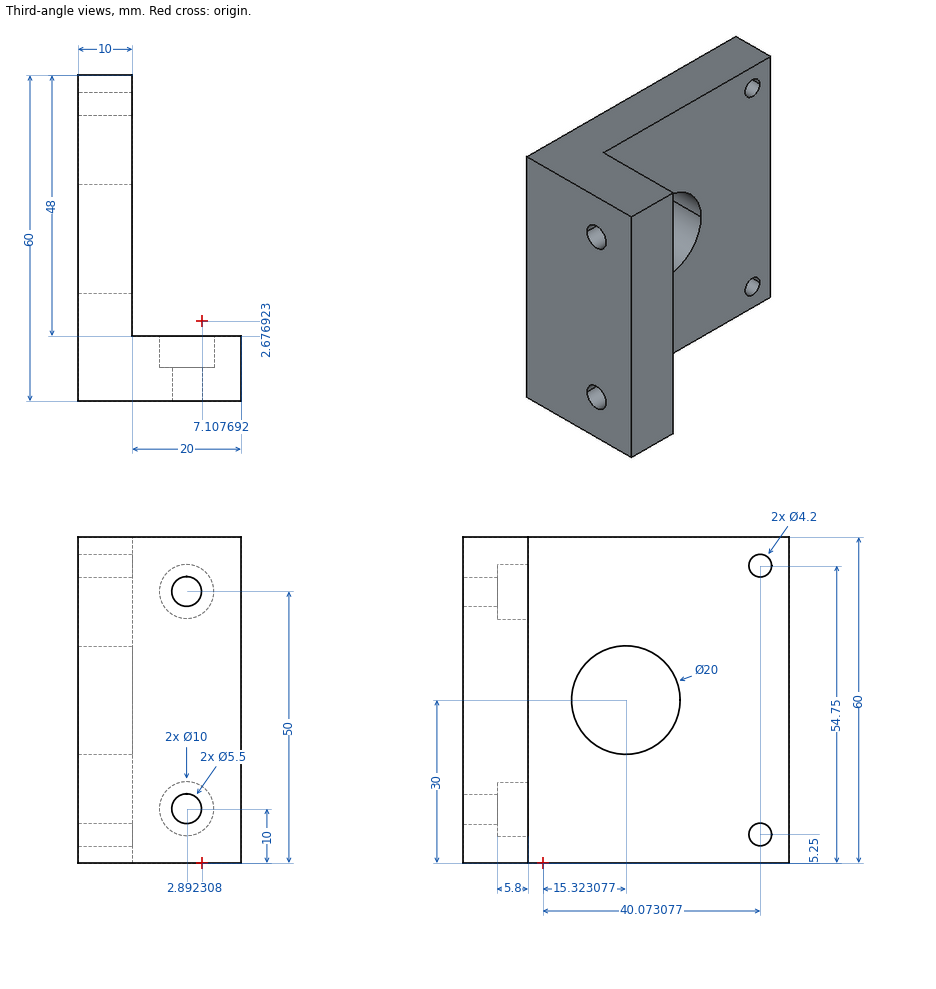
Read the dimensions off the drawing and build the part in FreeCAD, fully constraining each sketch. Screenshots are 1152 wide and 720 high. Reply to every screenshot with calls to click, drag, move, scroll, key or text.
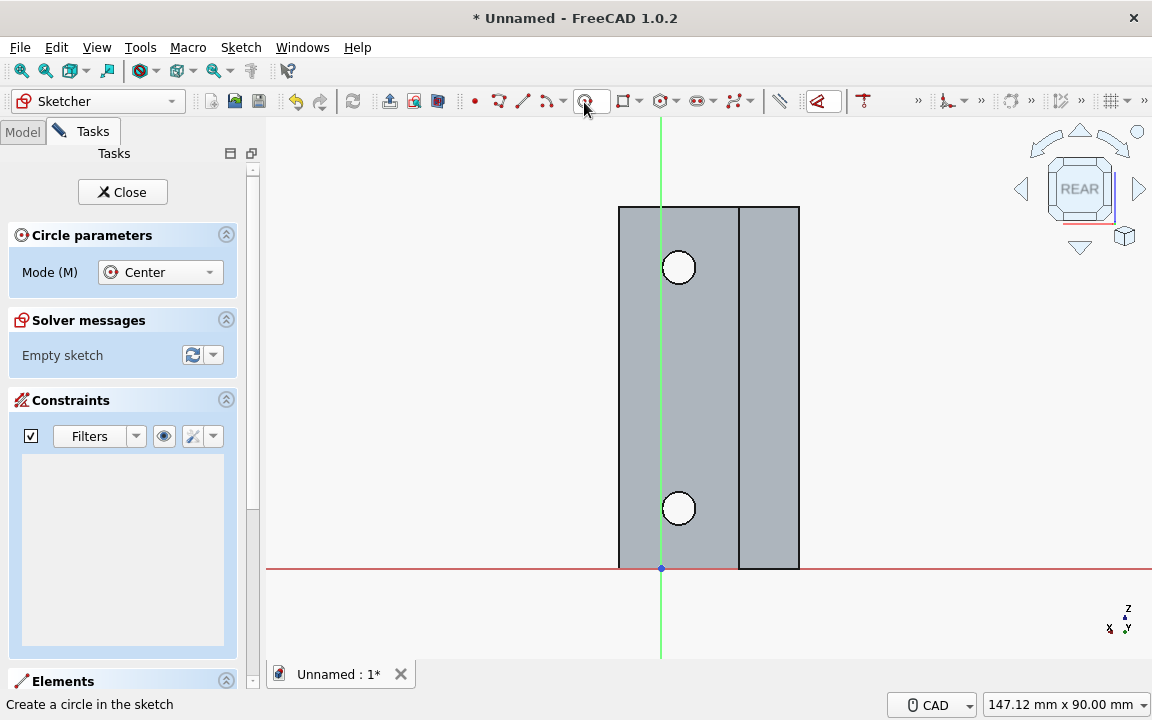
click(679, 508)
move(700, 487)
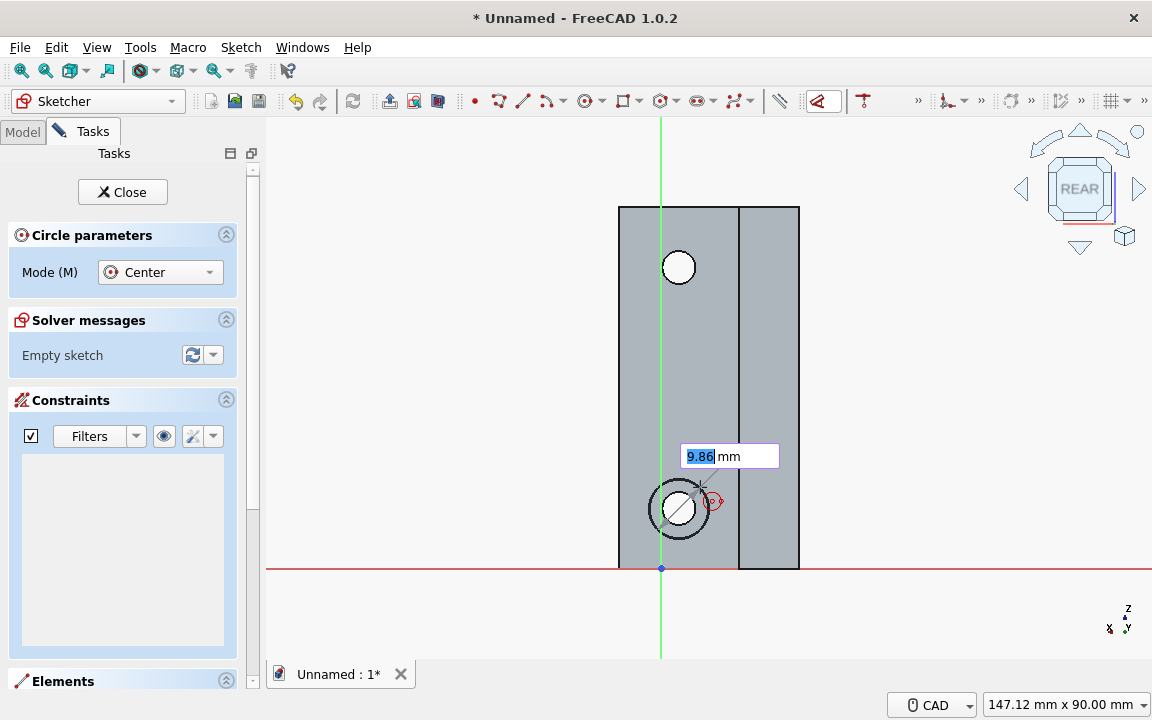
text(10)
key(Return)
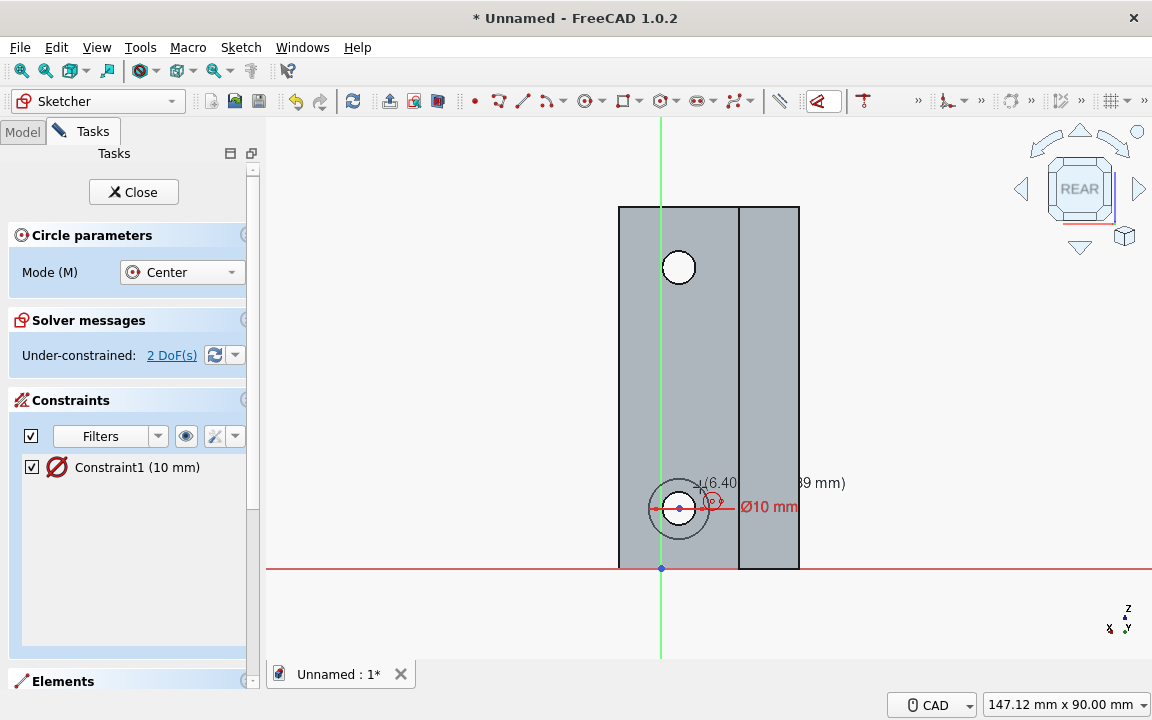
click(679, 268)
move(700, 246)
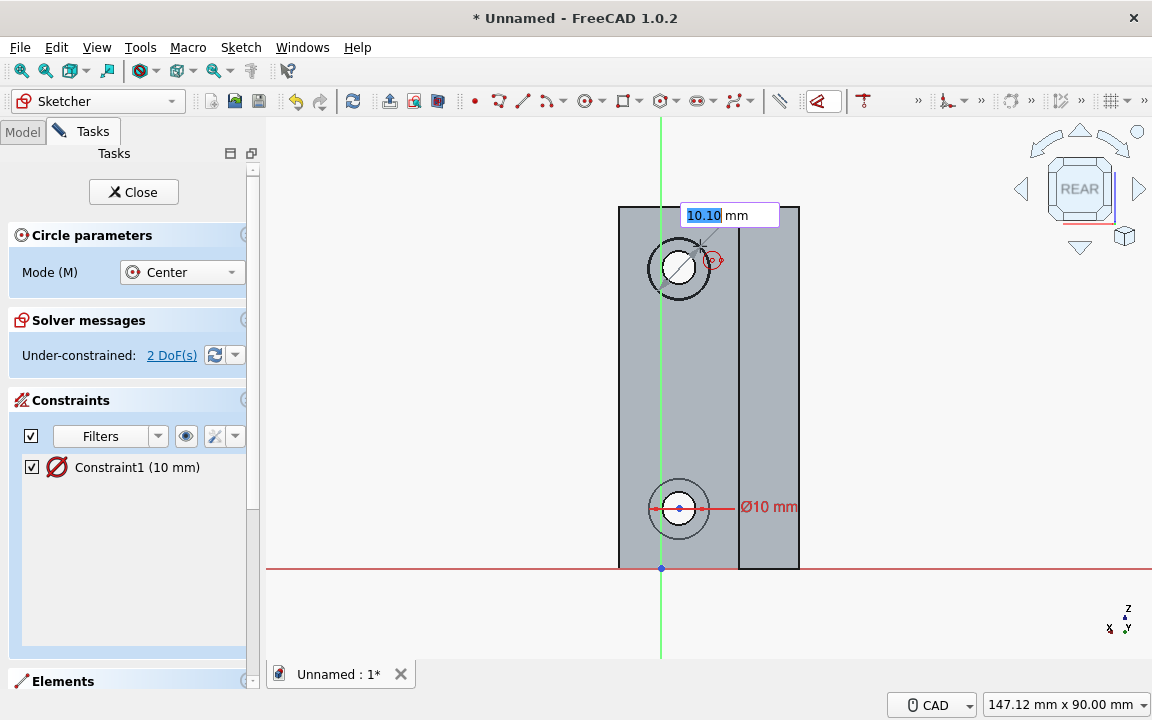
text(10)
key(Return)
key(Escape)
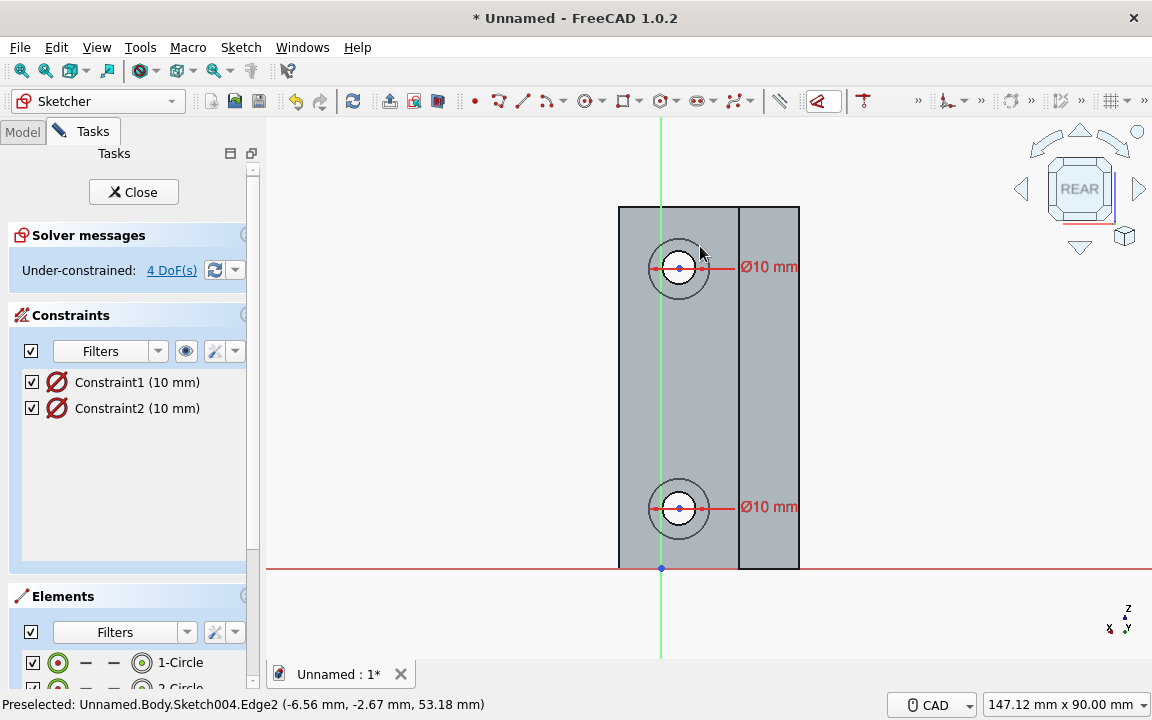
click(679, 509)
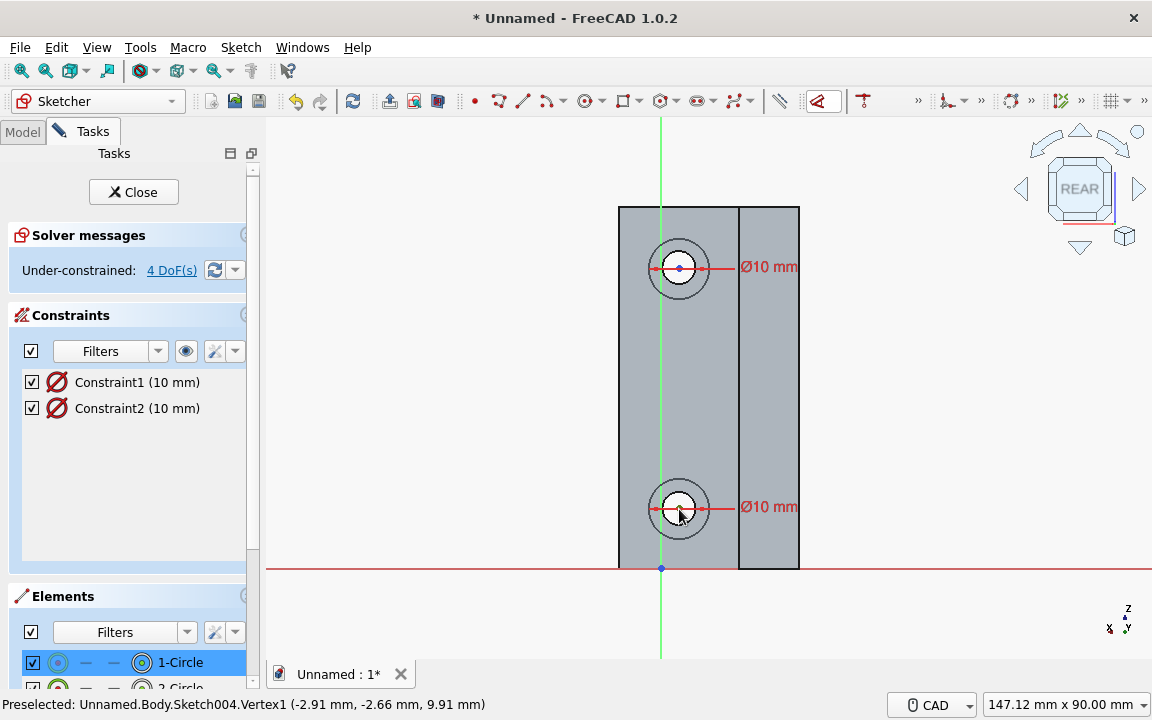
click(679, 269)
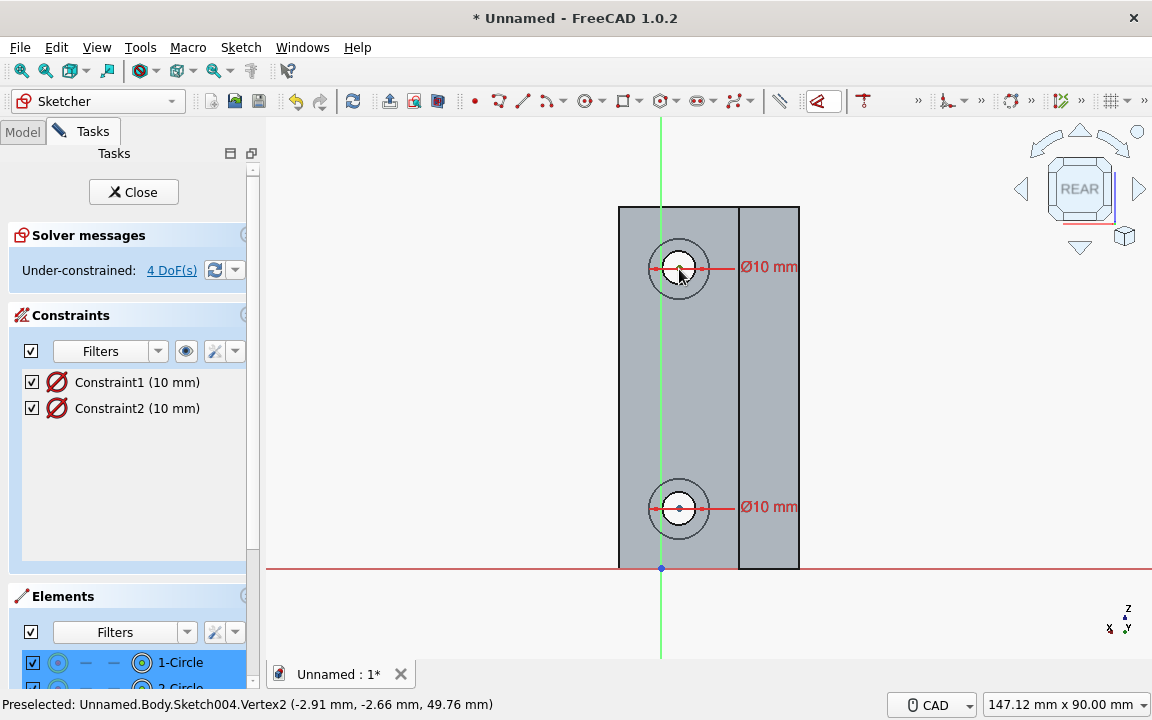
key(v)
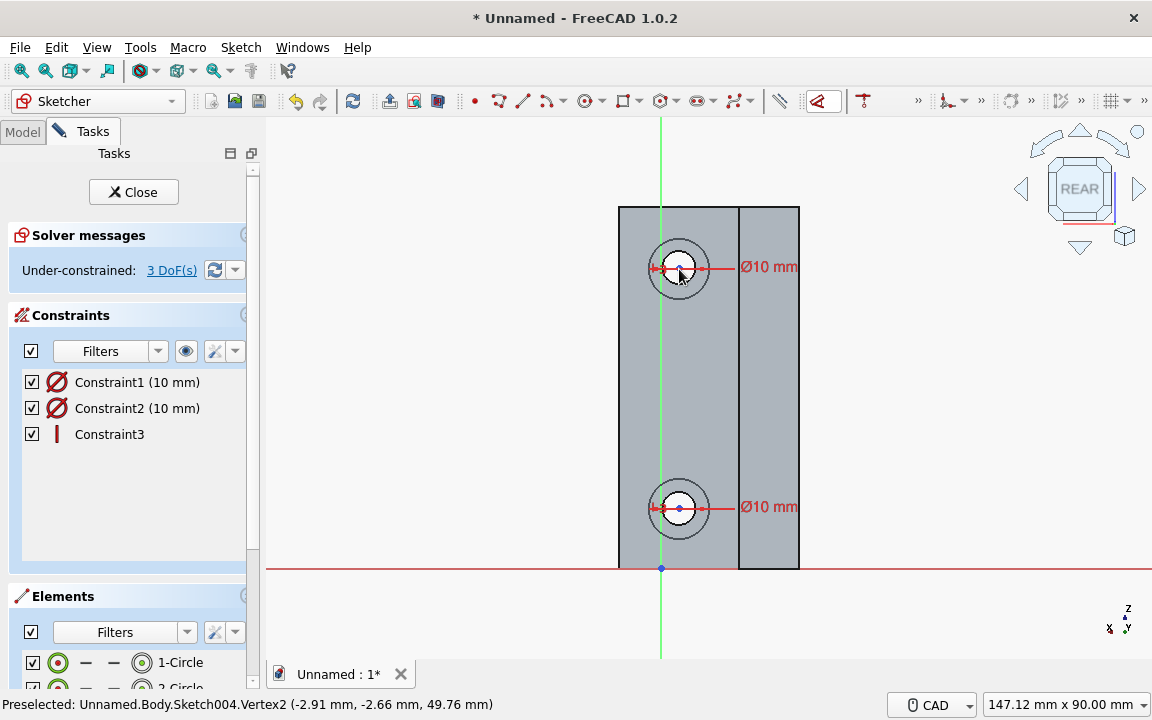
click(679, 509)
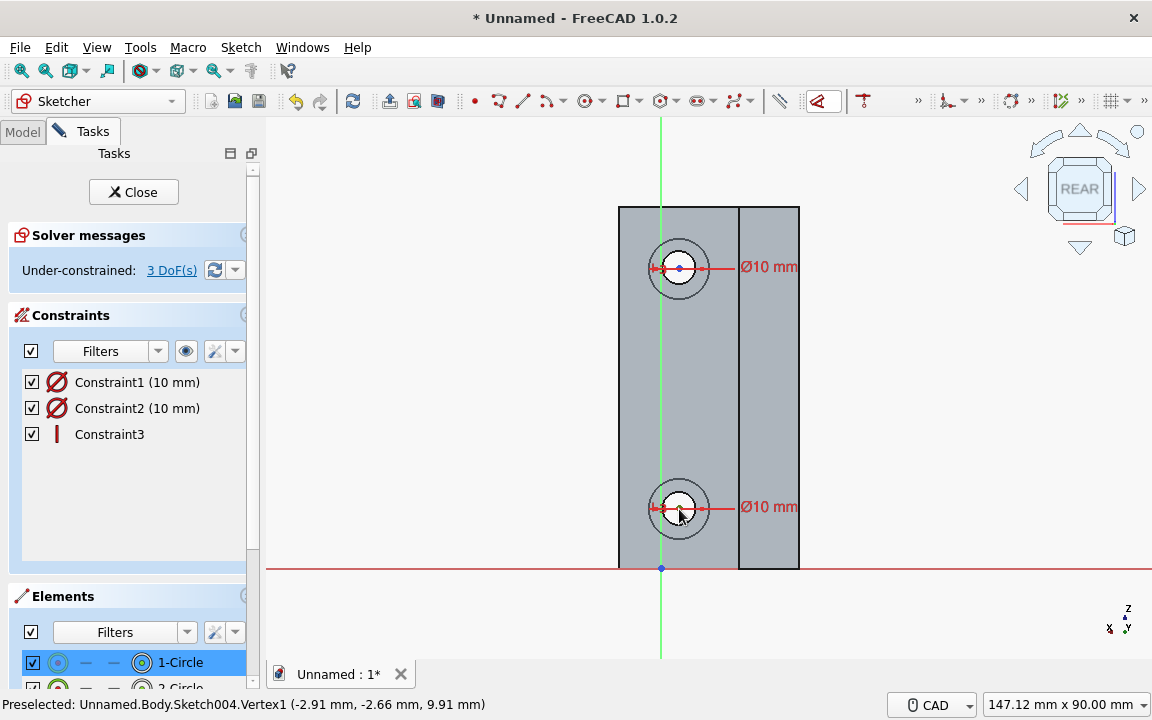
key(i)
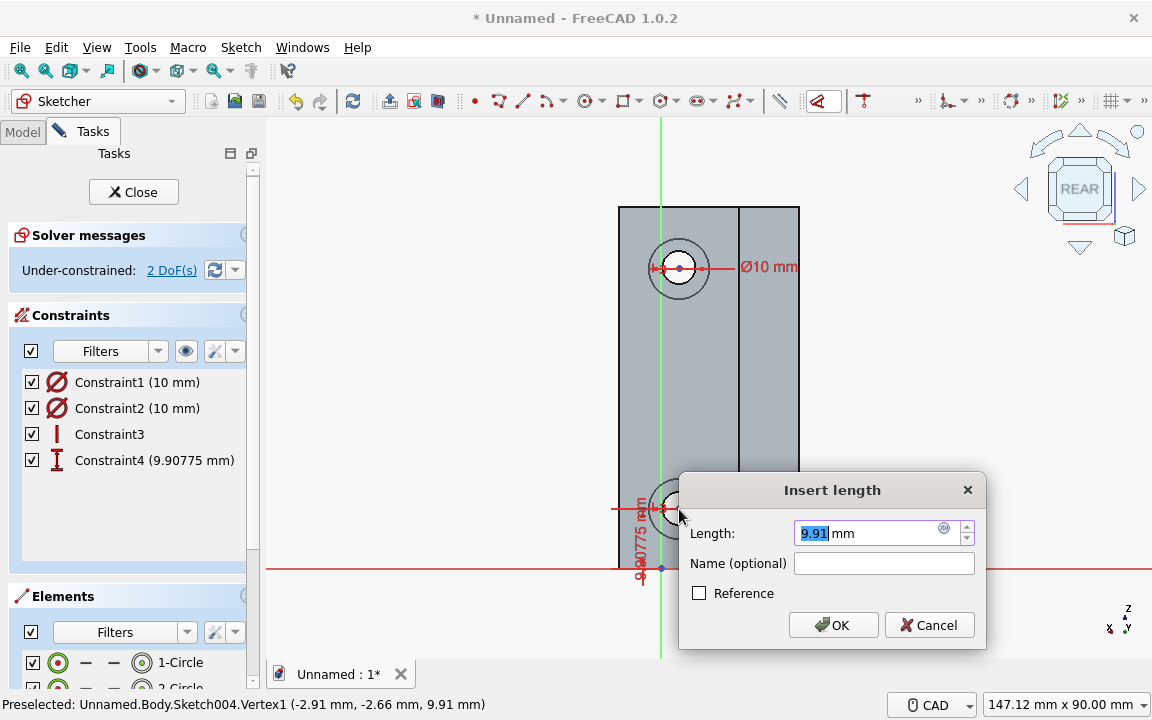
text(10)
key(Return)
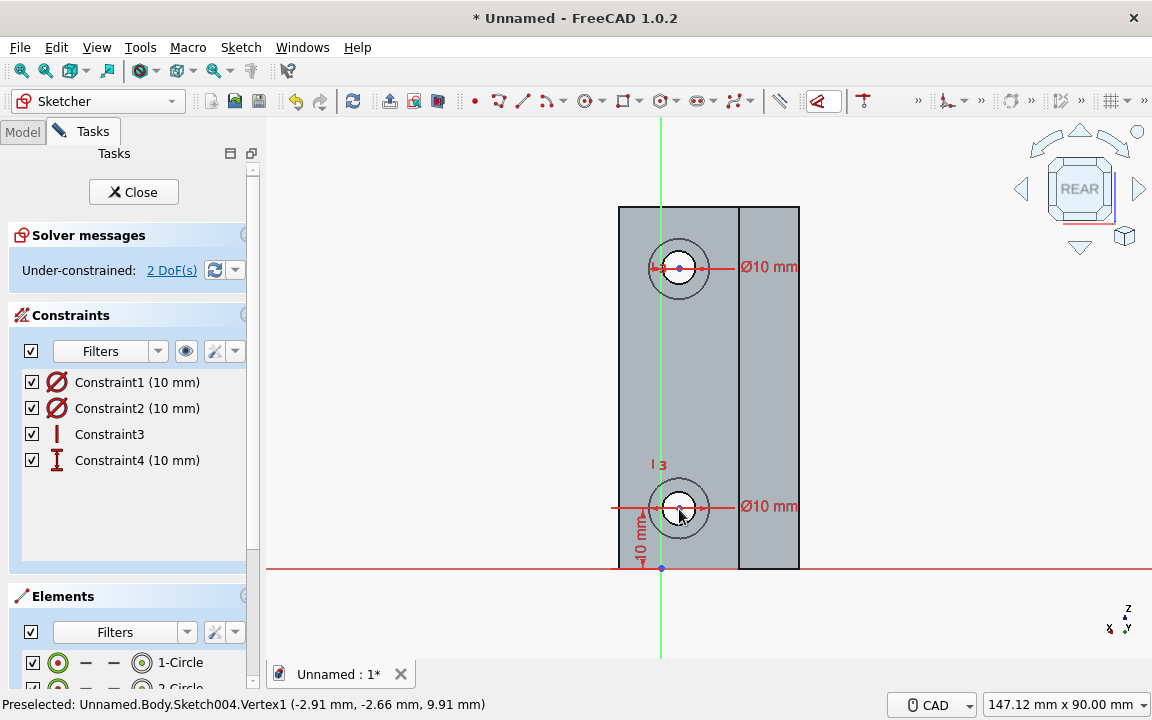
click(679, 269)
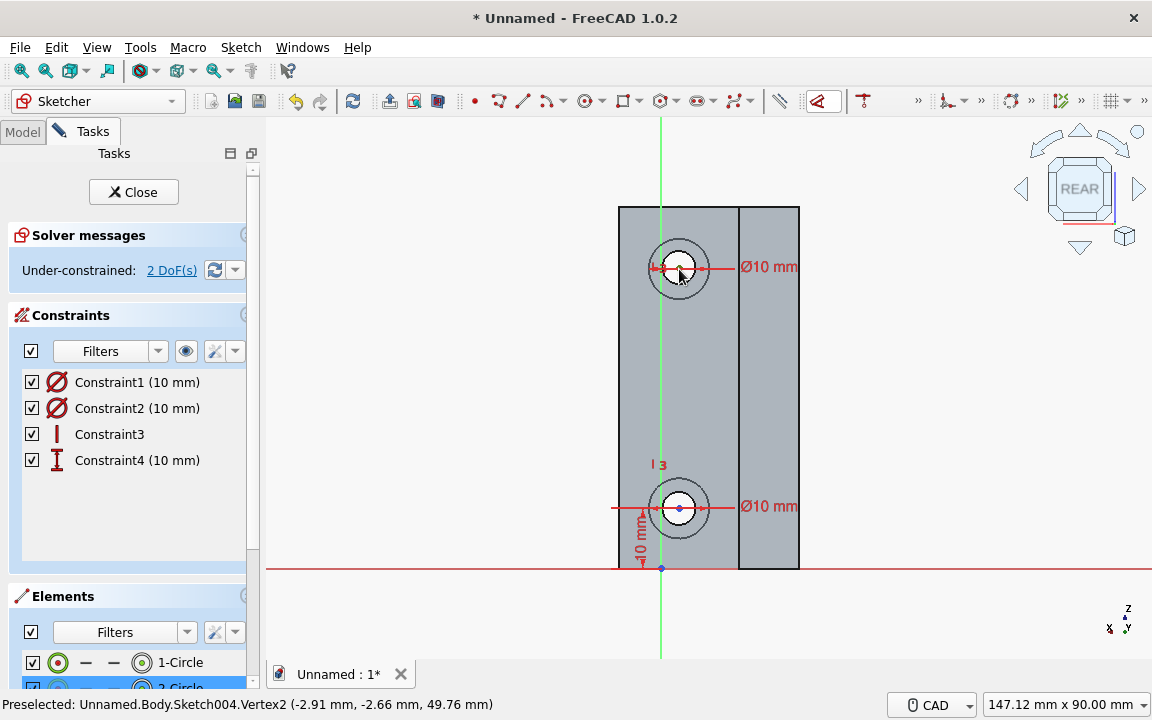
key(i)